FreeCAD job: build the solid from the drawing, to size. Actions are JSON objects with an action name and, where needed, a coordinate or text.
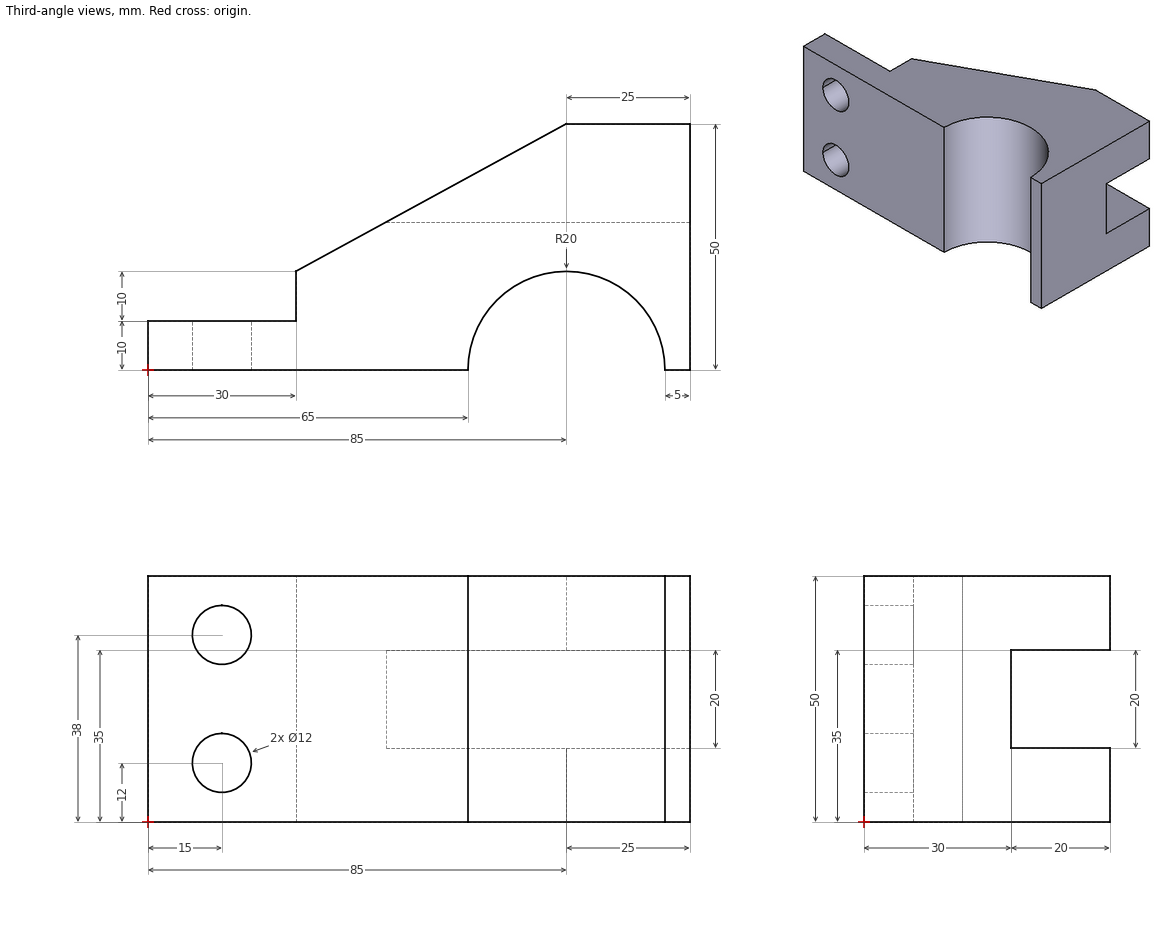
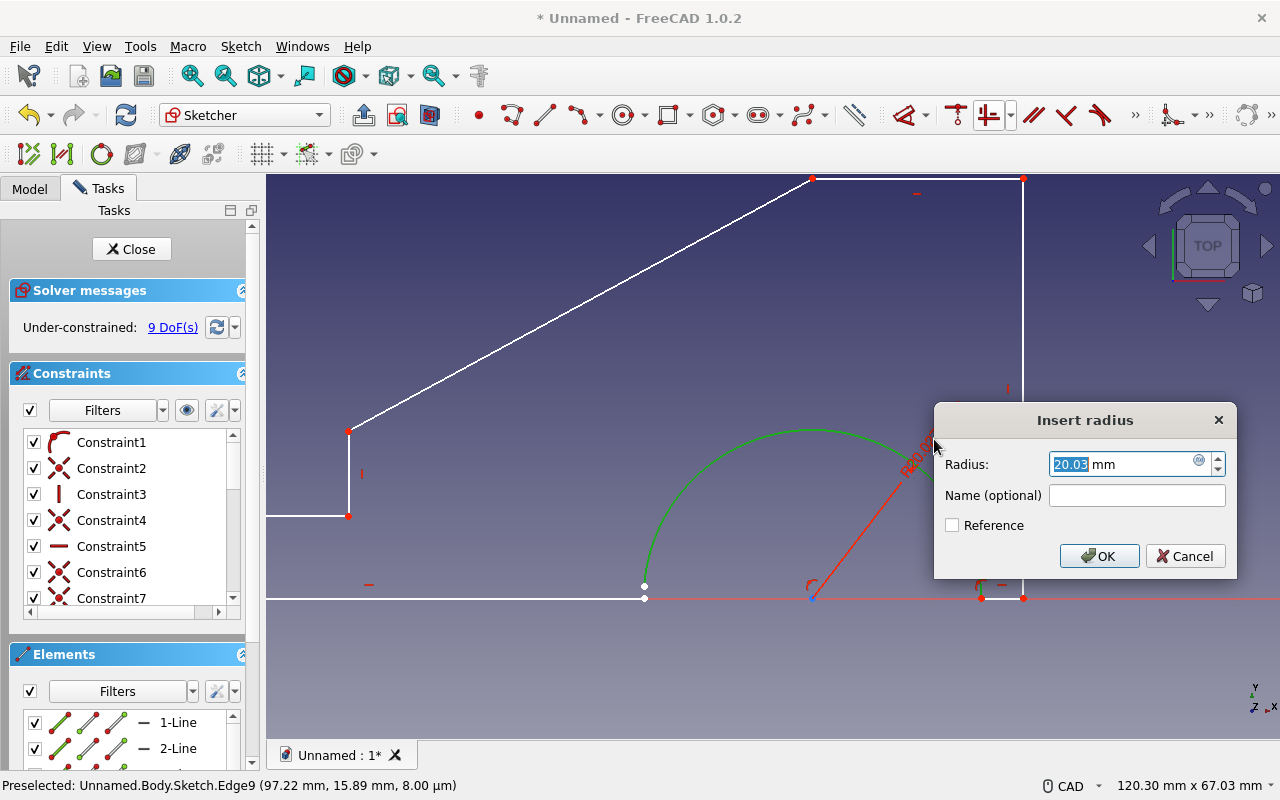
{"action": "type", "text": "20"}
{"action": "key", "text": "Return"}
{"action": "key", "text": "Escape"}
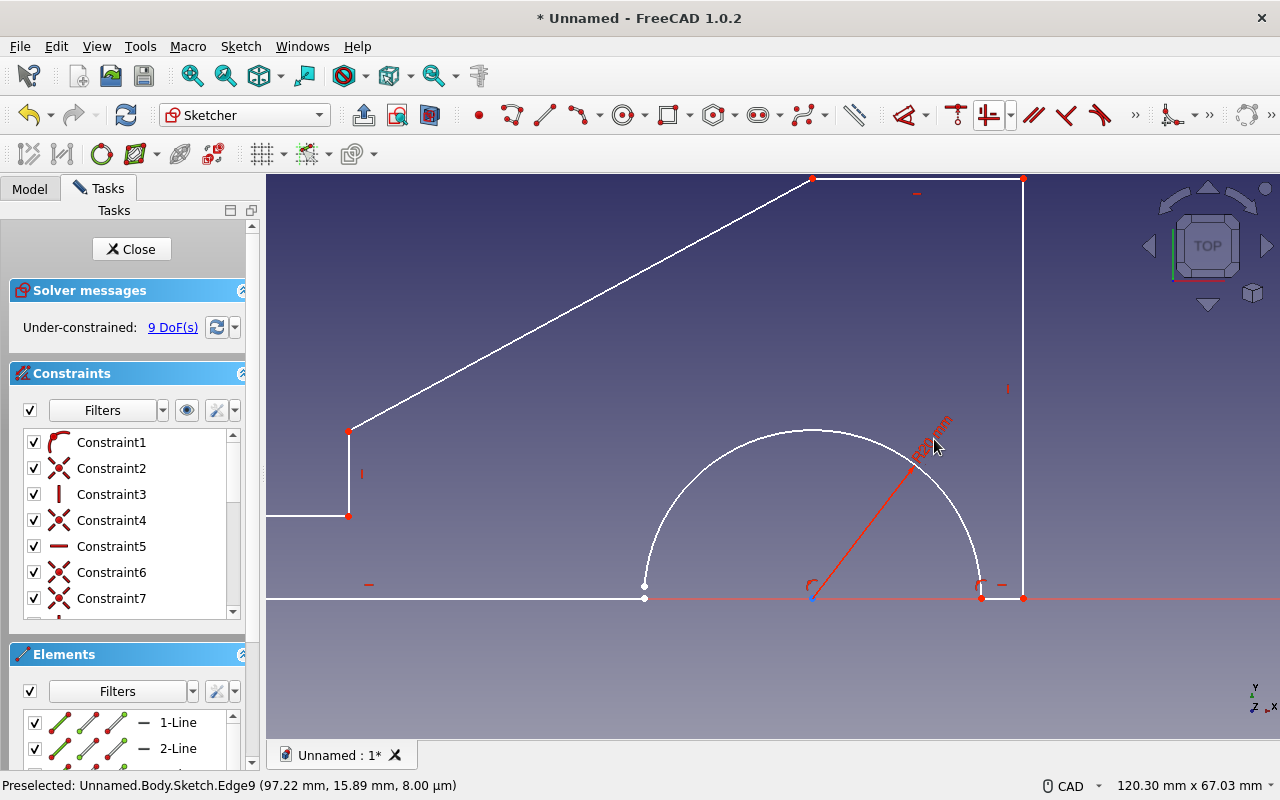
{"action": "left_click", "coordinate": [645, 586]}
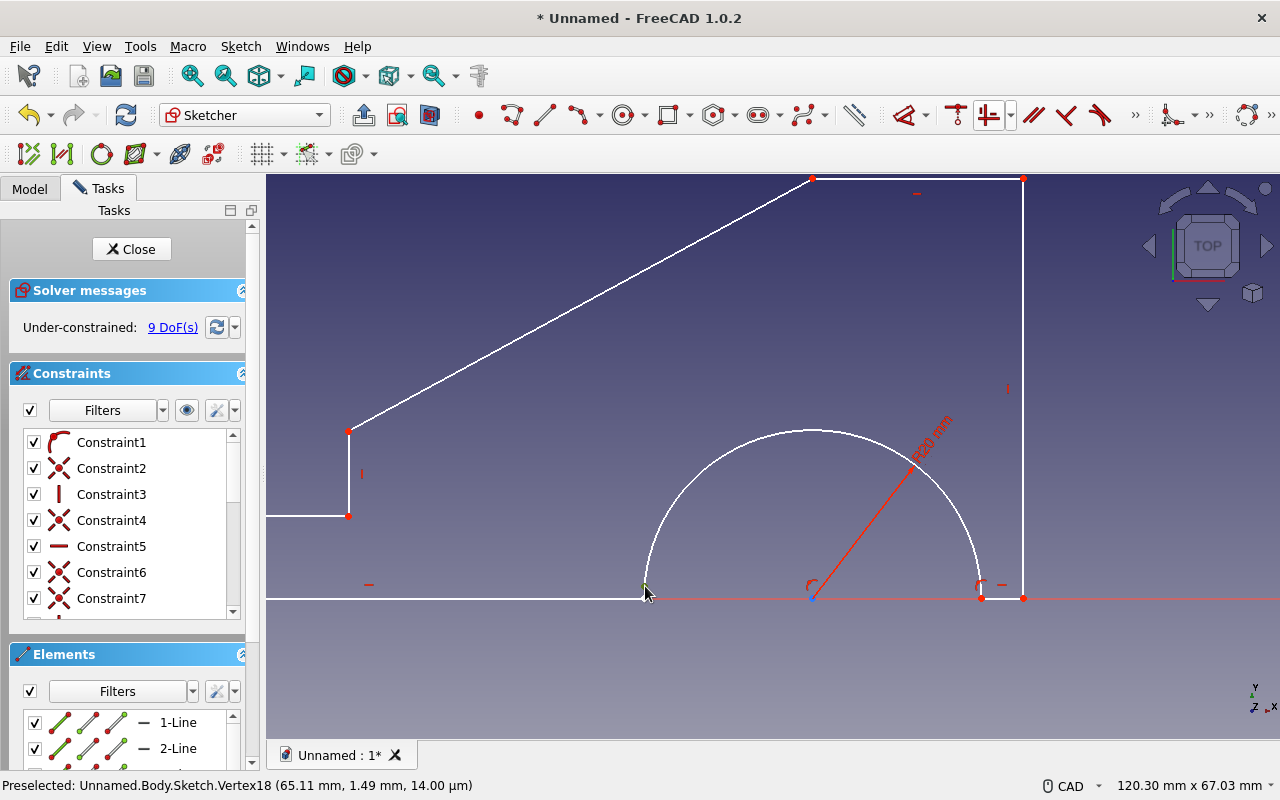
{"action": "left_click", "coordinate": [704, 599]}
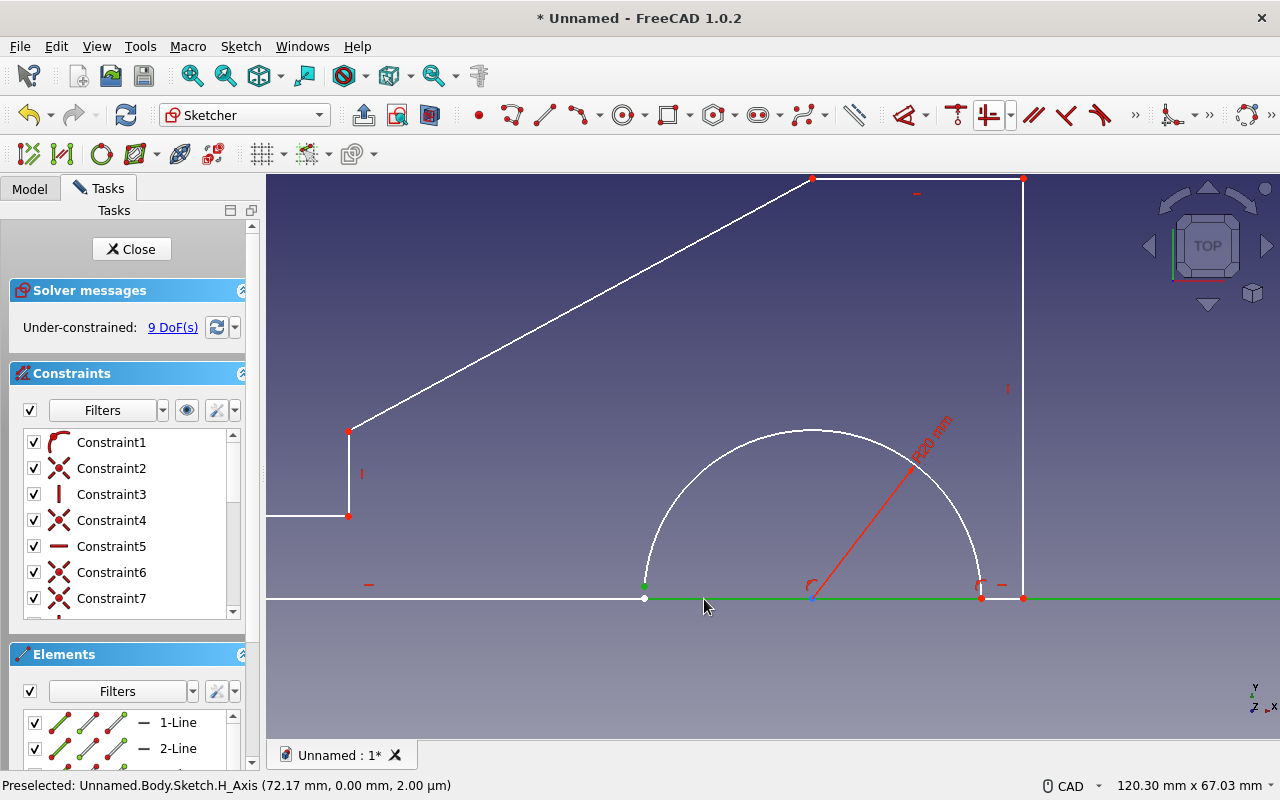
{"action": "left_click", "coordinate": [956, 116]}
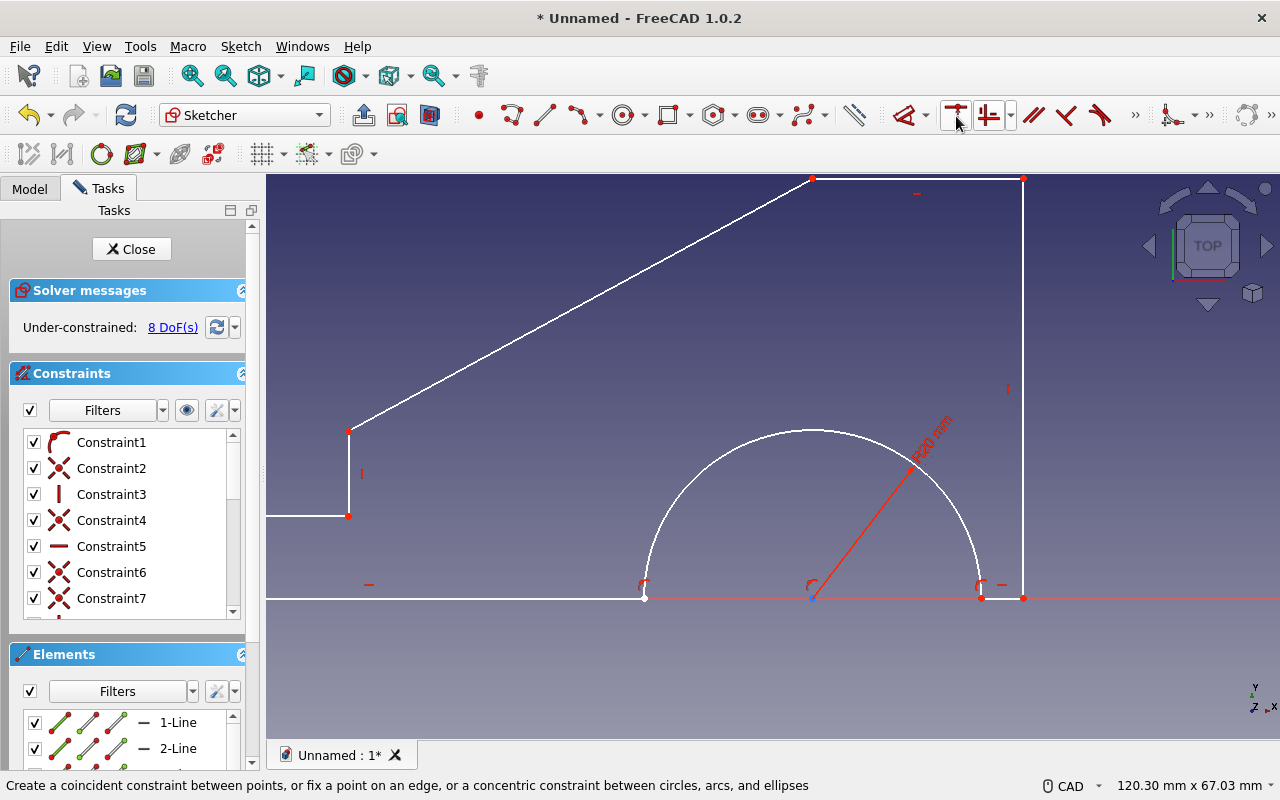
{"action": "left_click", "coordinate": [904, 116]}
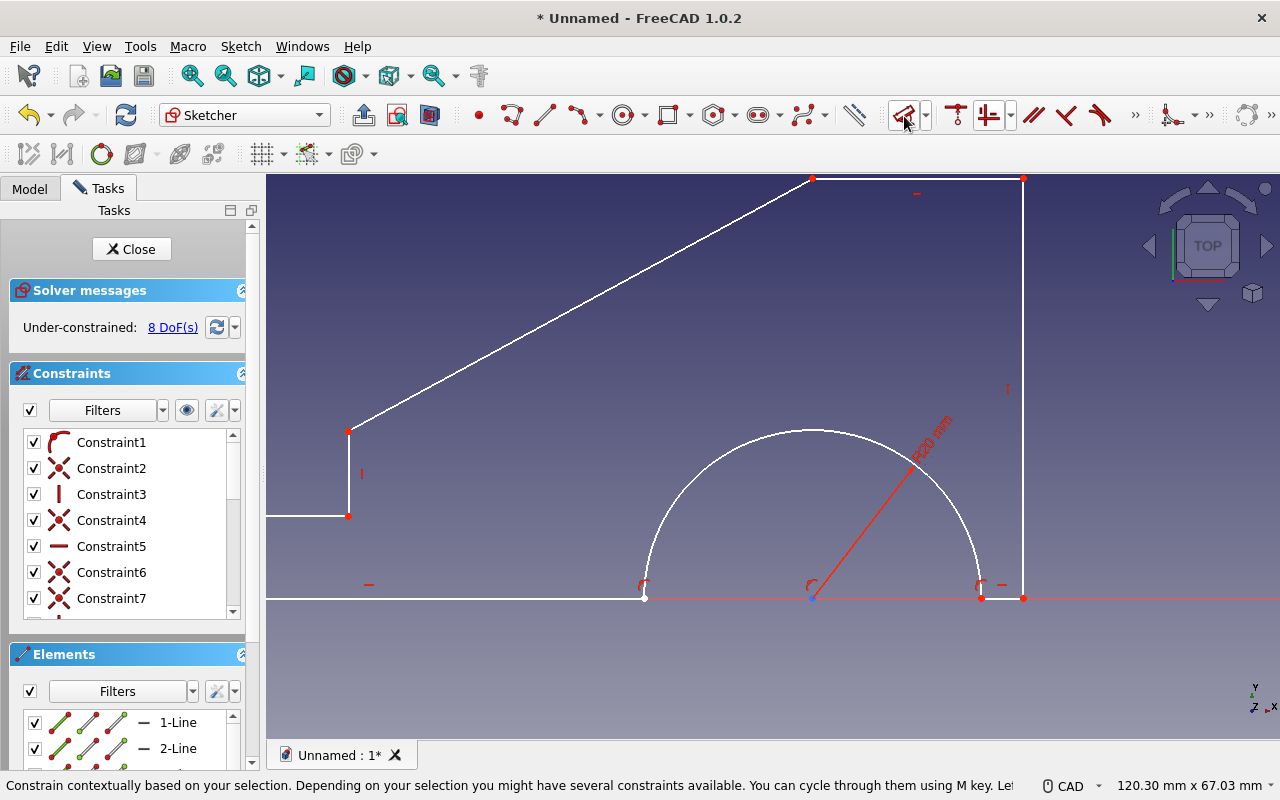
{"action": "left_click", "coordinate": [994, 599]}
{"action": "left_click", "coordinate": [1002, 633]}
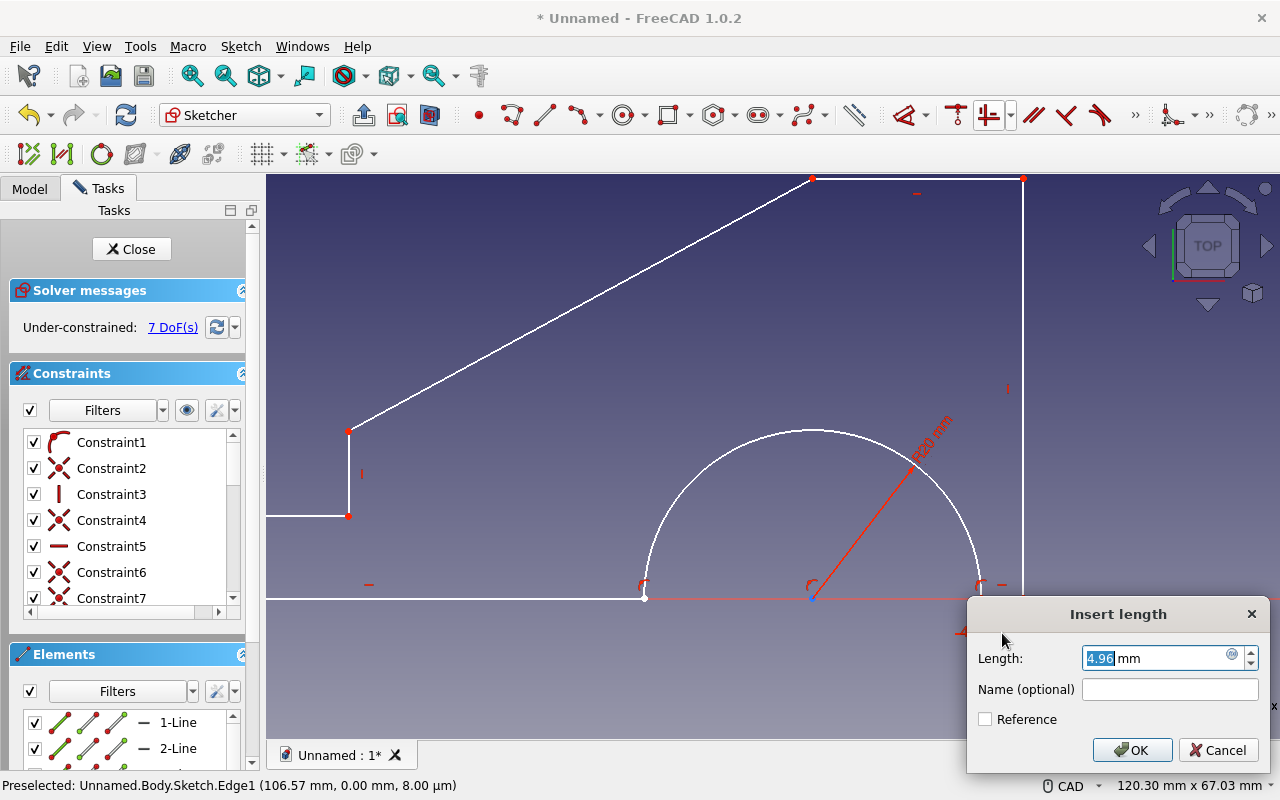
{"action": "type", "text": "5"}
{"action": "key", "text": "Return"}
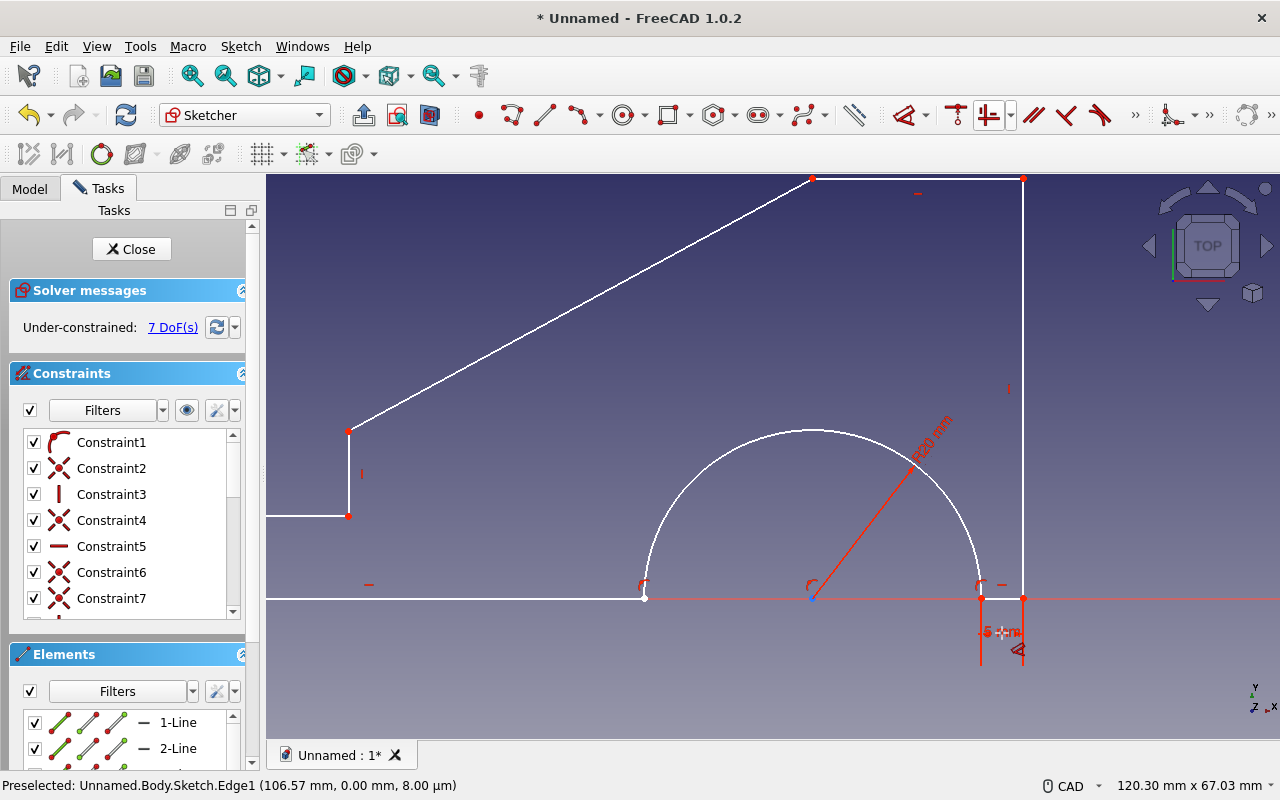
{"action": "left_click", "coordinate": [1023, 473]}
{"action": "left_click", "coordinate": [1057, 400]}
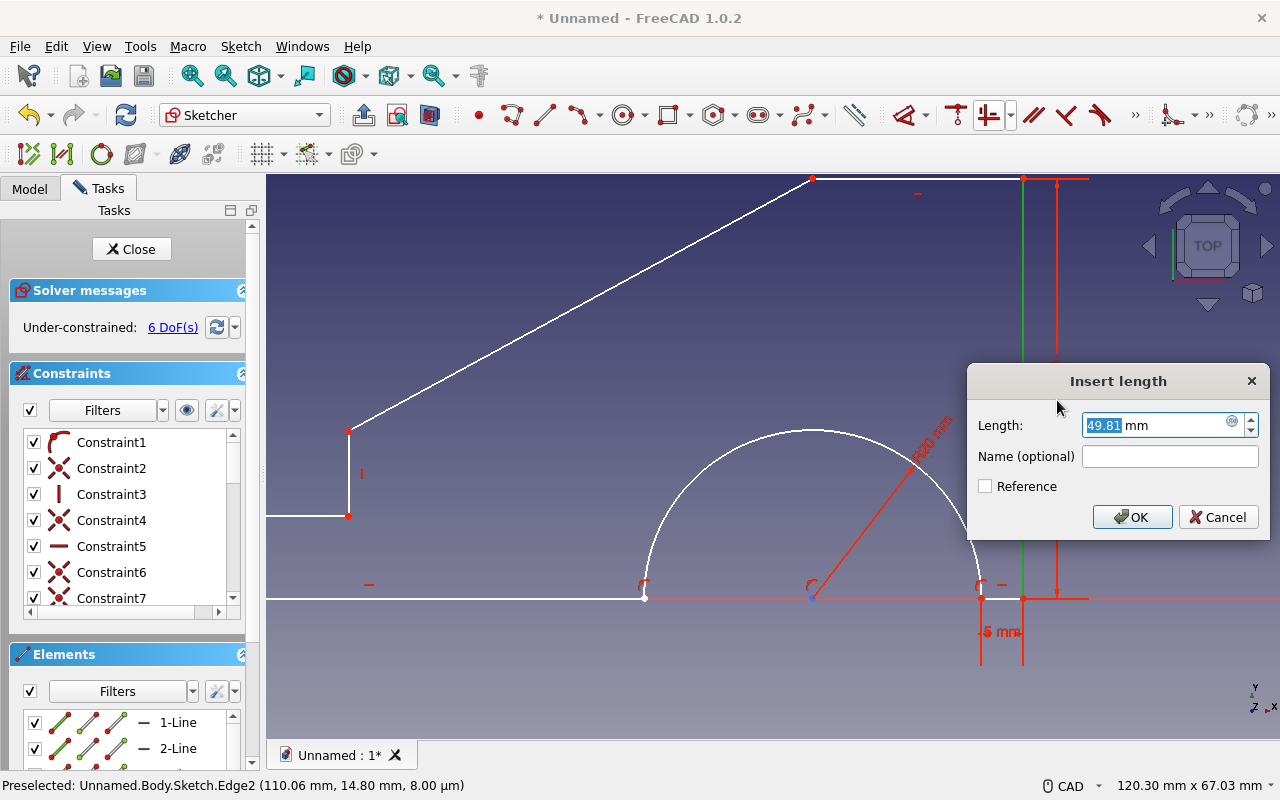
{"action": "type", "text": "50"}
{"action": "key", "text": "Return"}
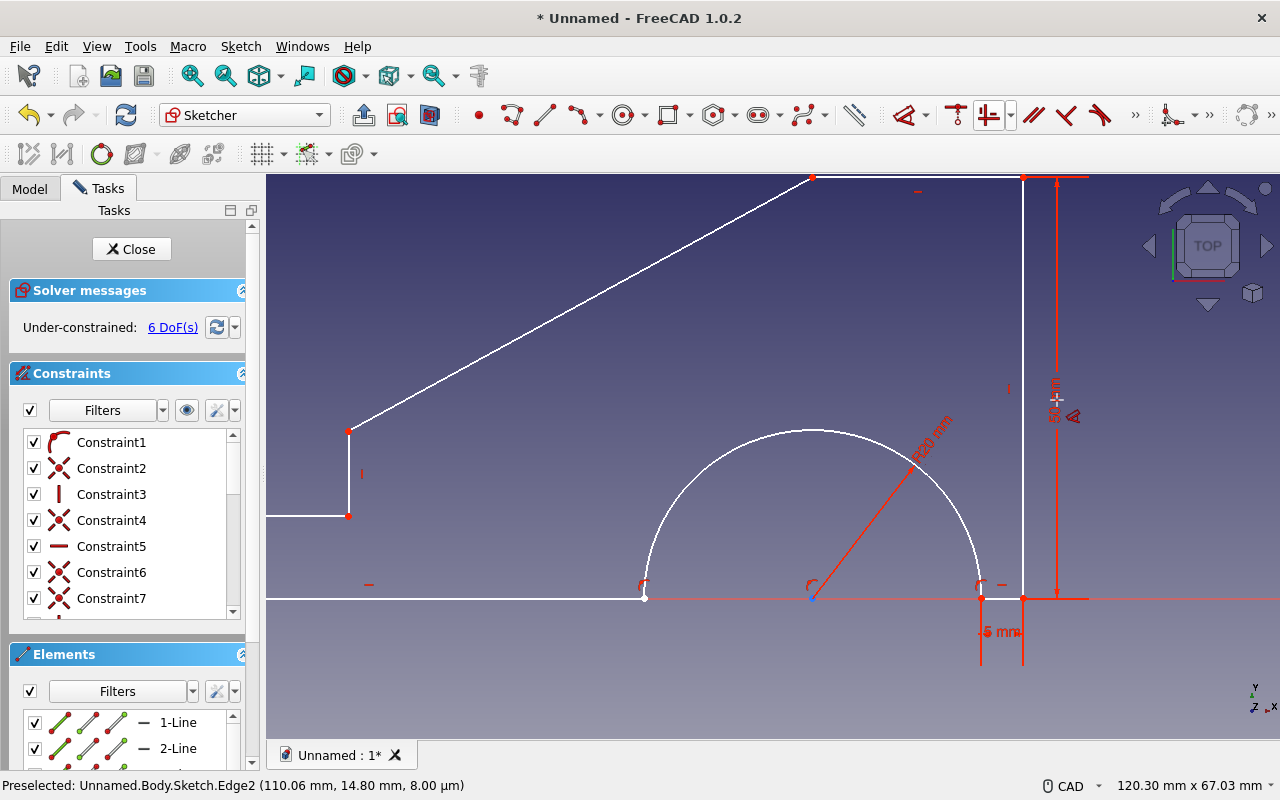
{"action": "scroll", "coordinate": [1000, 596], "scroll_direction": "down", "scroll_amount": 2}